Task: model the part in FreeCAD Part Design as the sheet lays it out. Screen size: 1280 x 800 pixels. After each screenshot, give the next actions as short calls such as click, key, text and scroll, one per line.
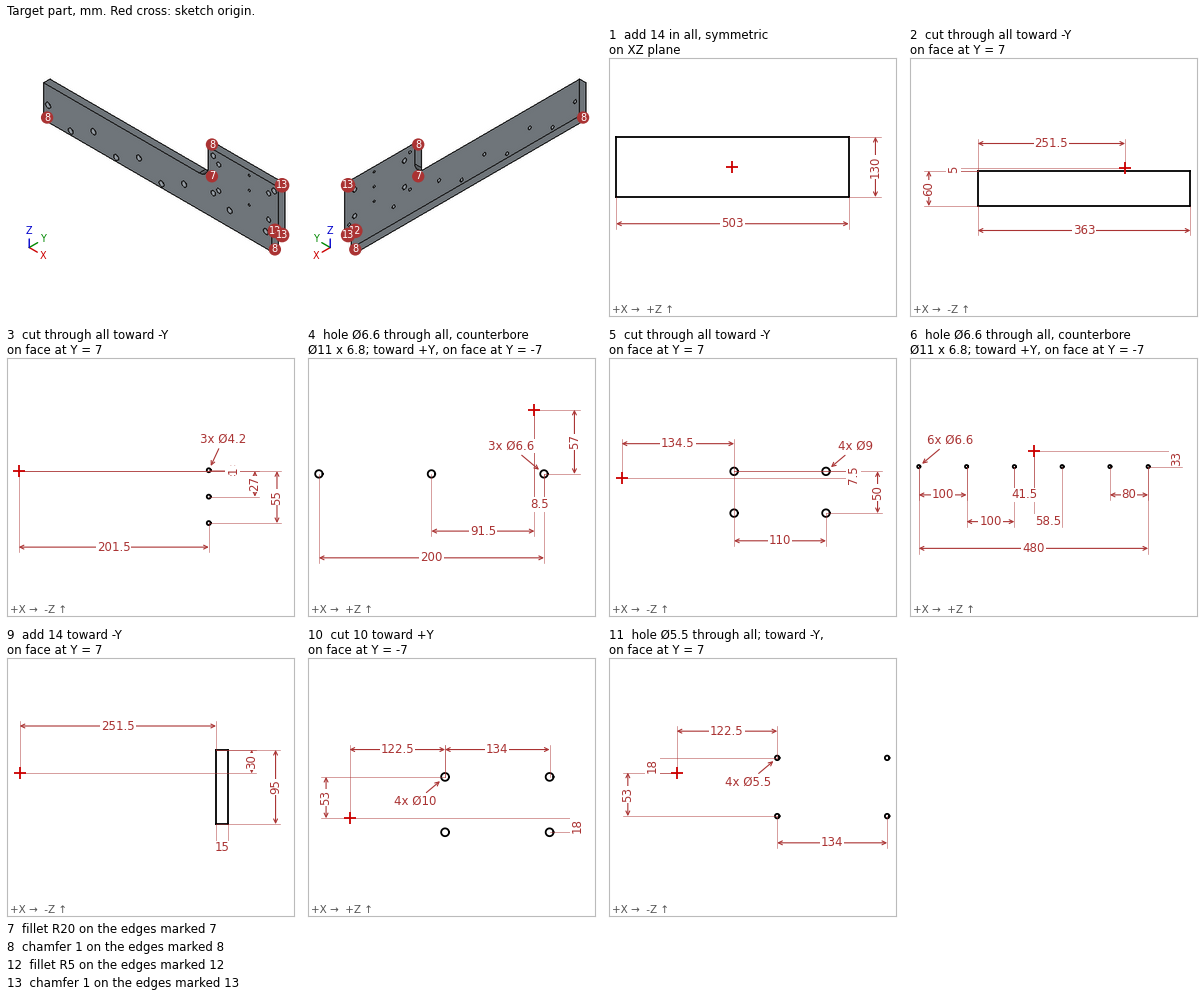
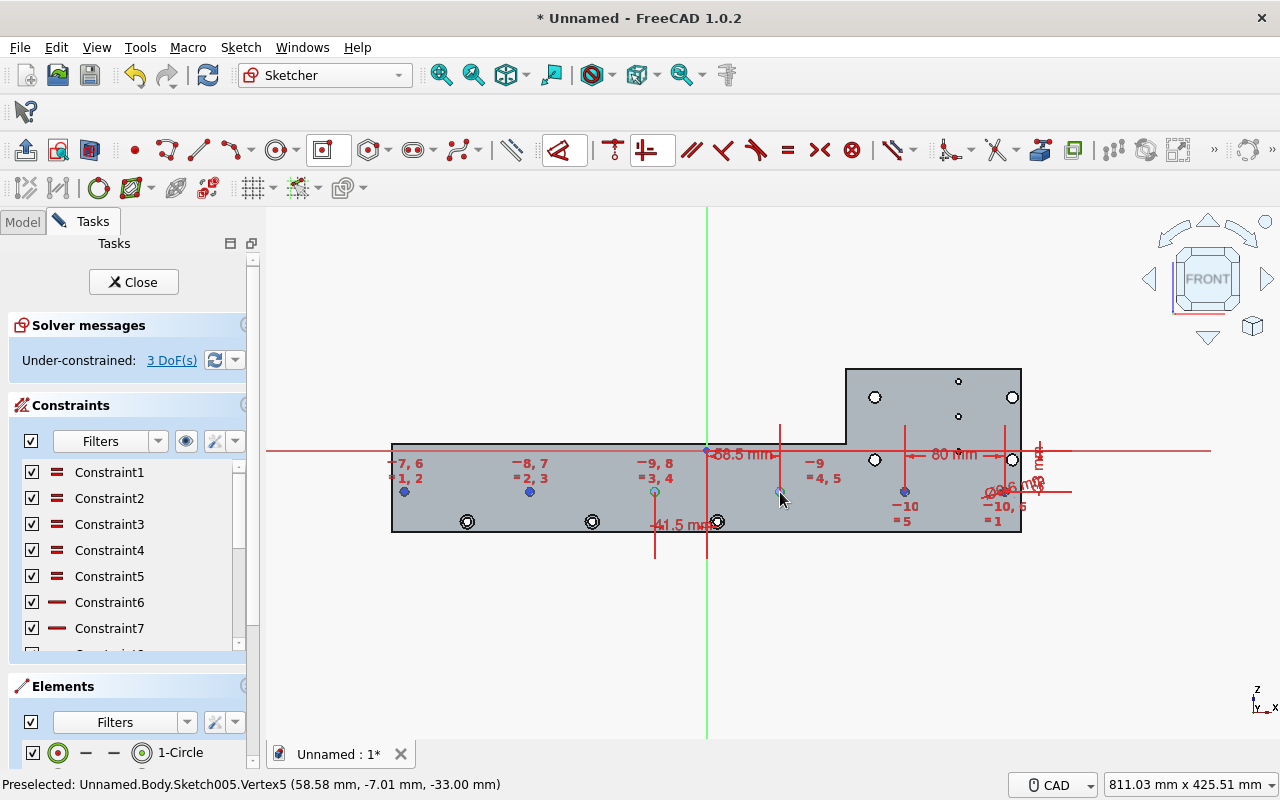
click(1005, 492)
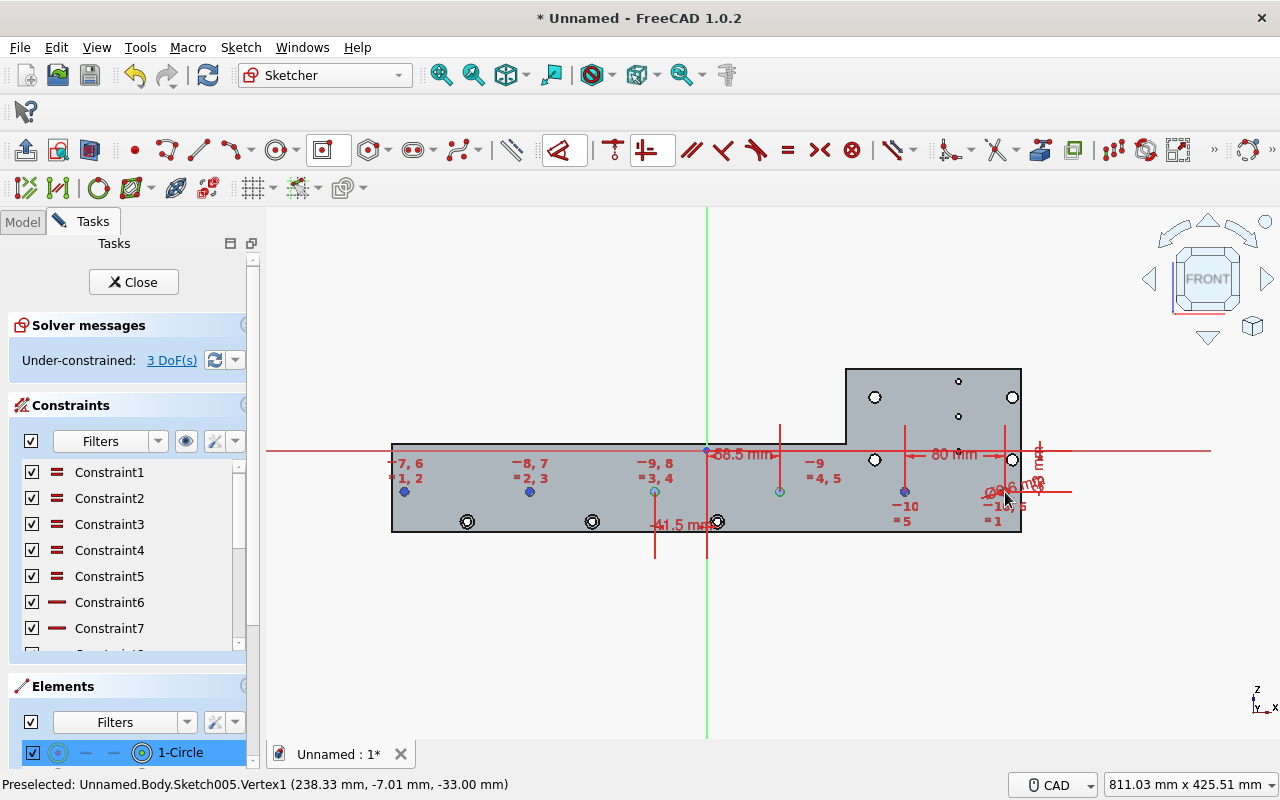
click(404, 492)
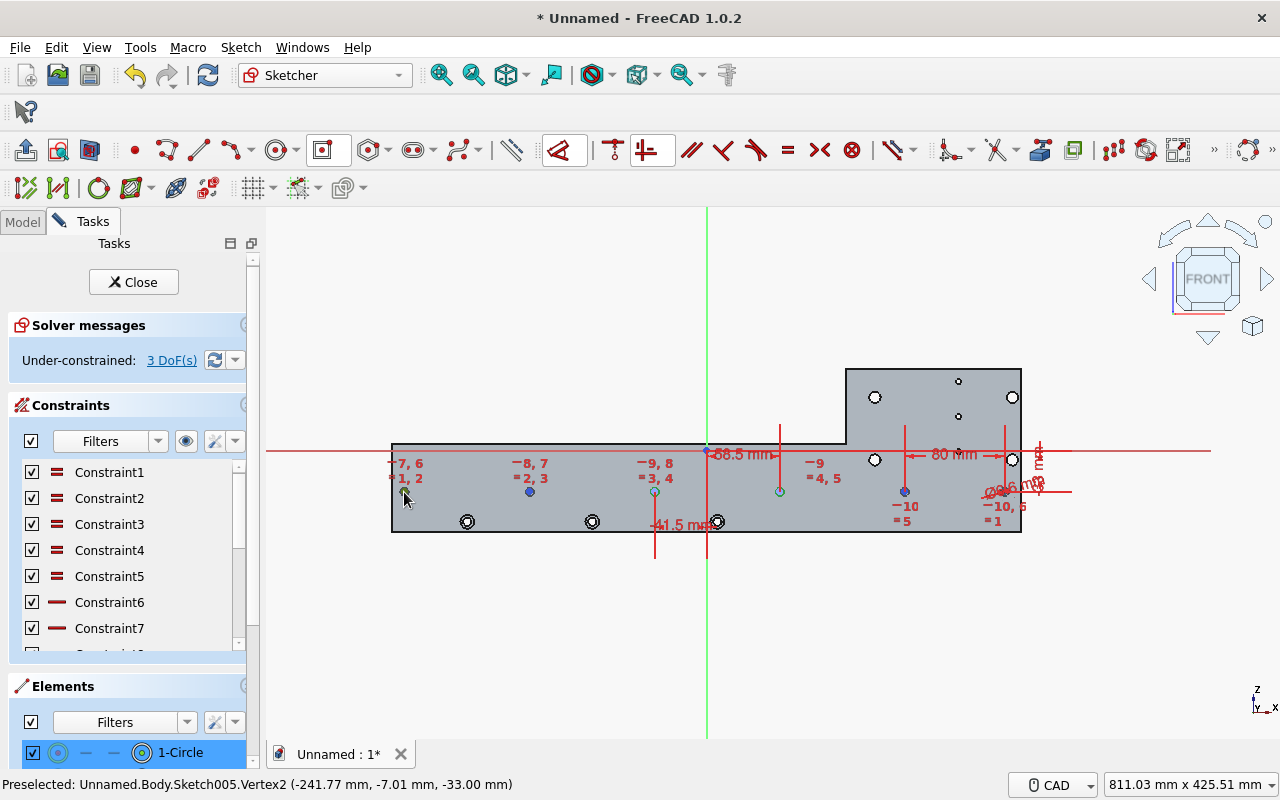
key(l)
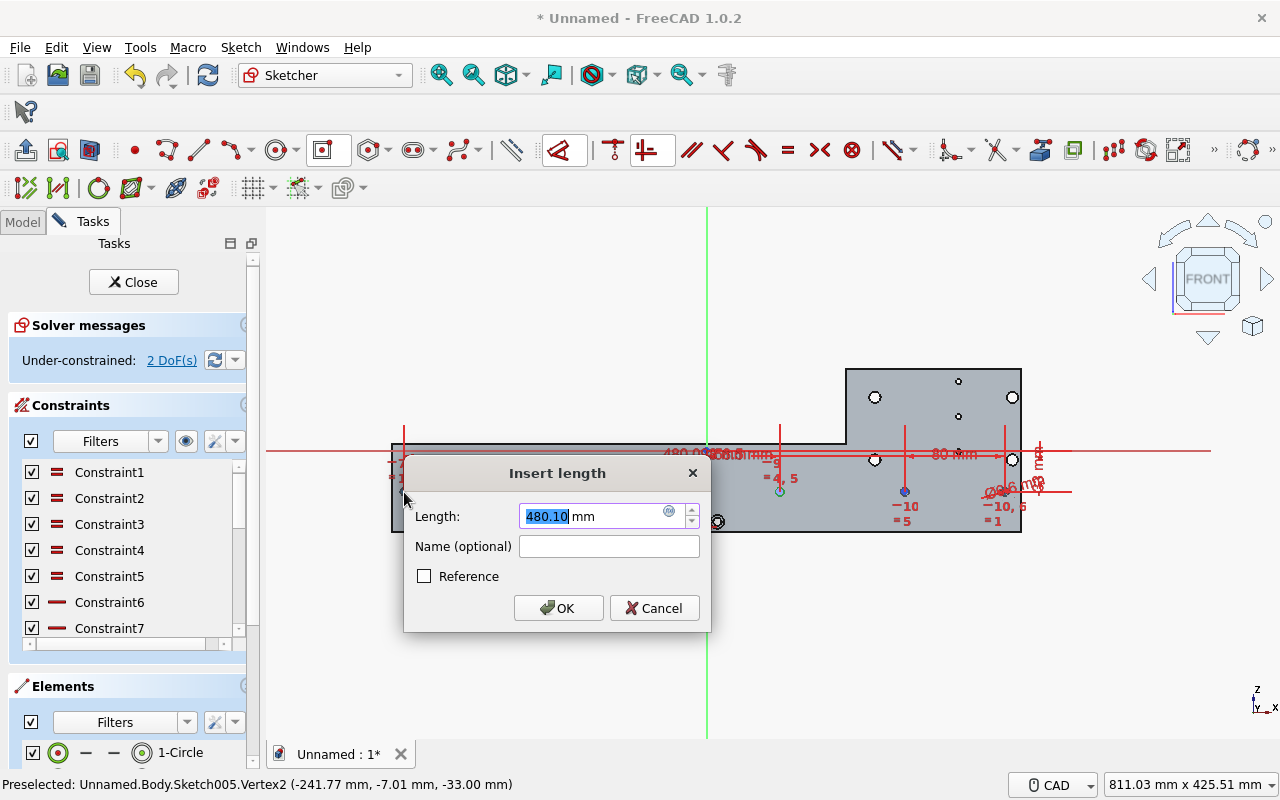
text(480)
key(Return)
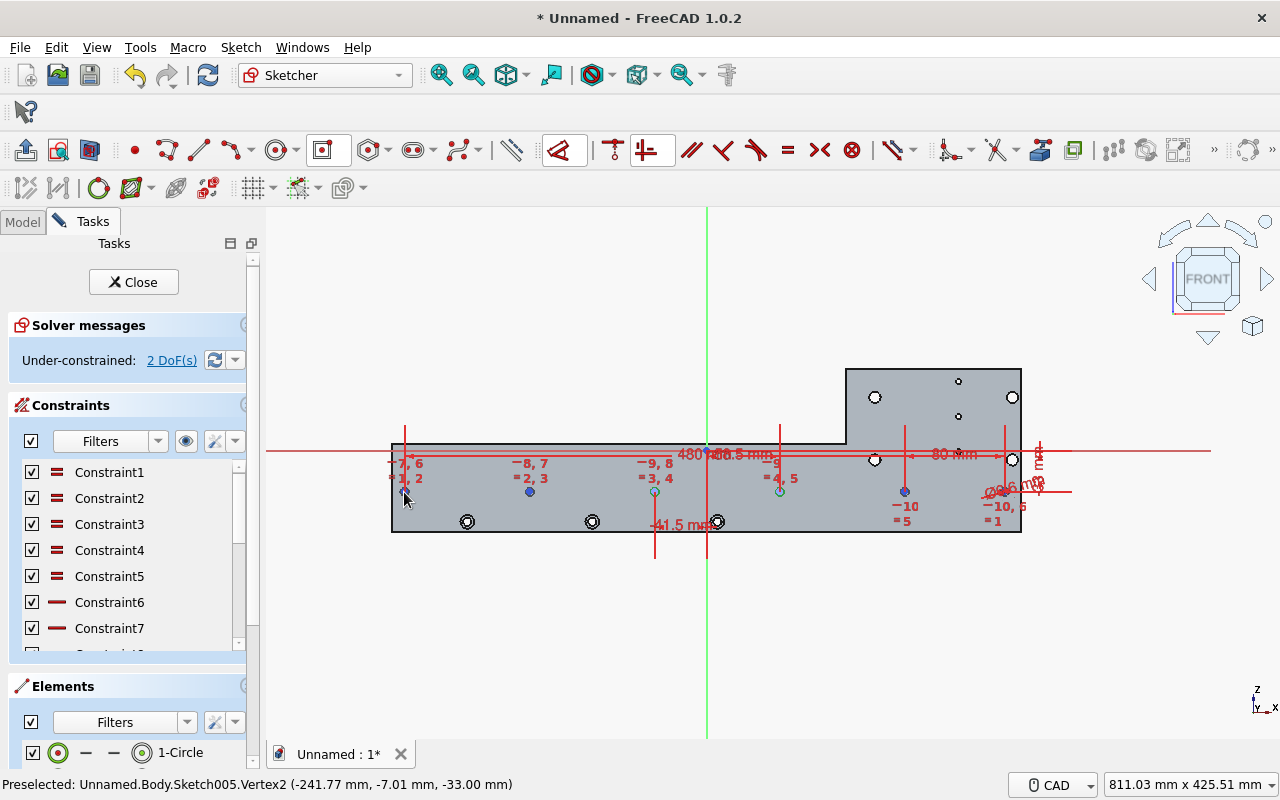
click(405, 492)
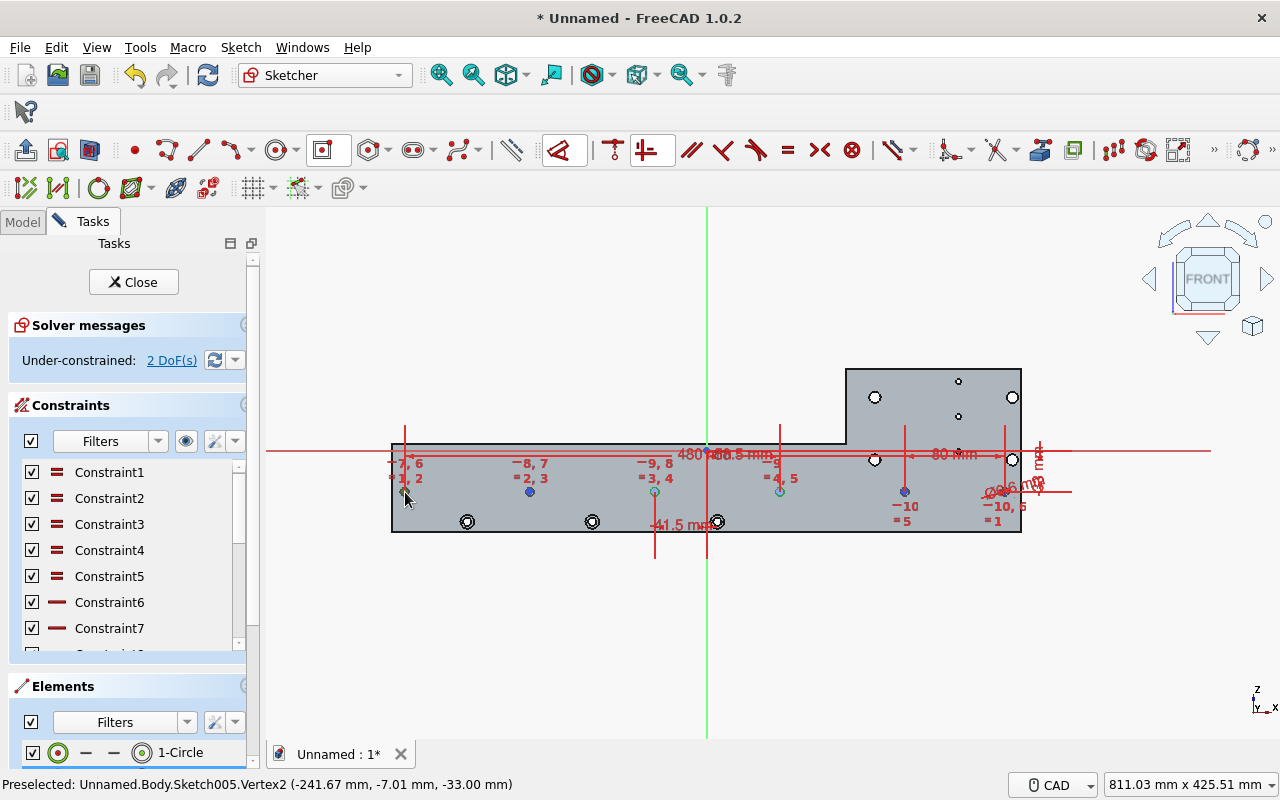
click(530, 492)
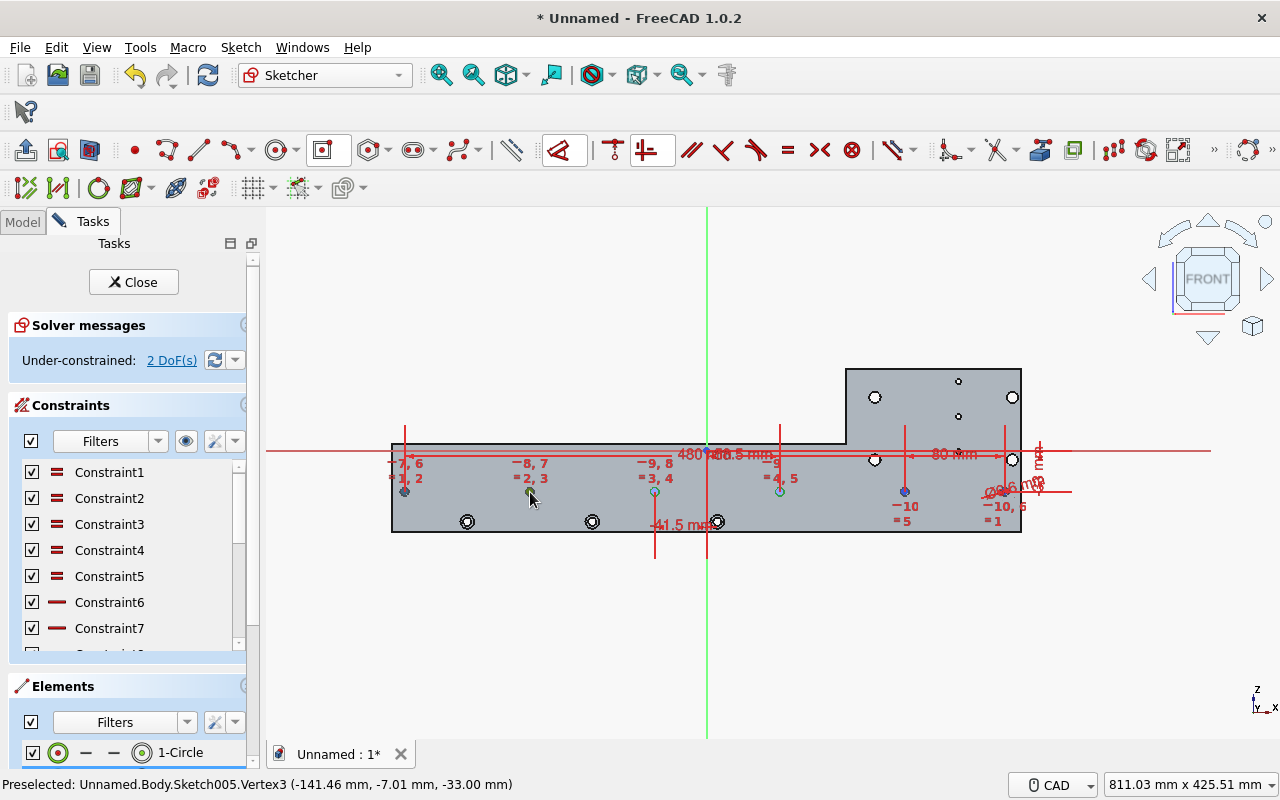
key(l)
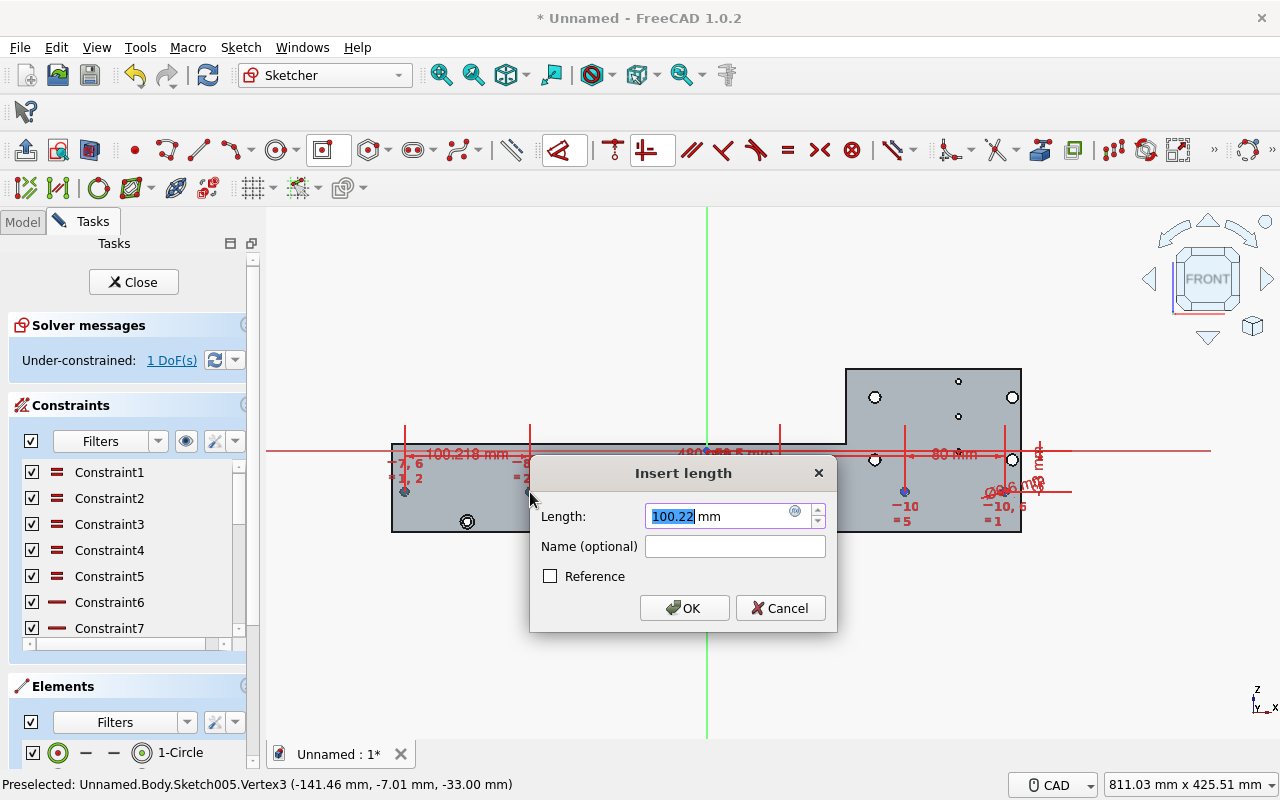
text(100)
key(Return)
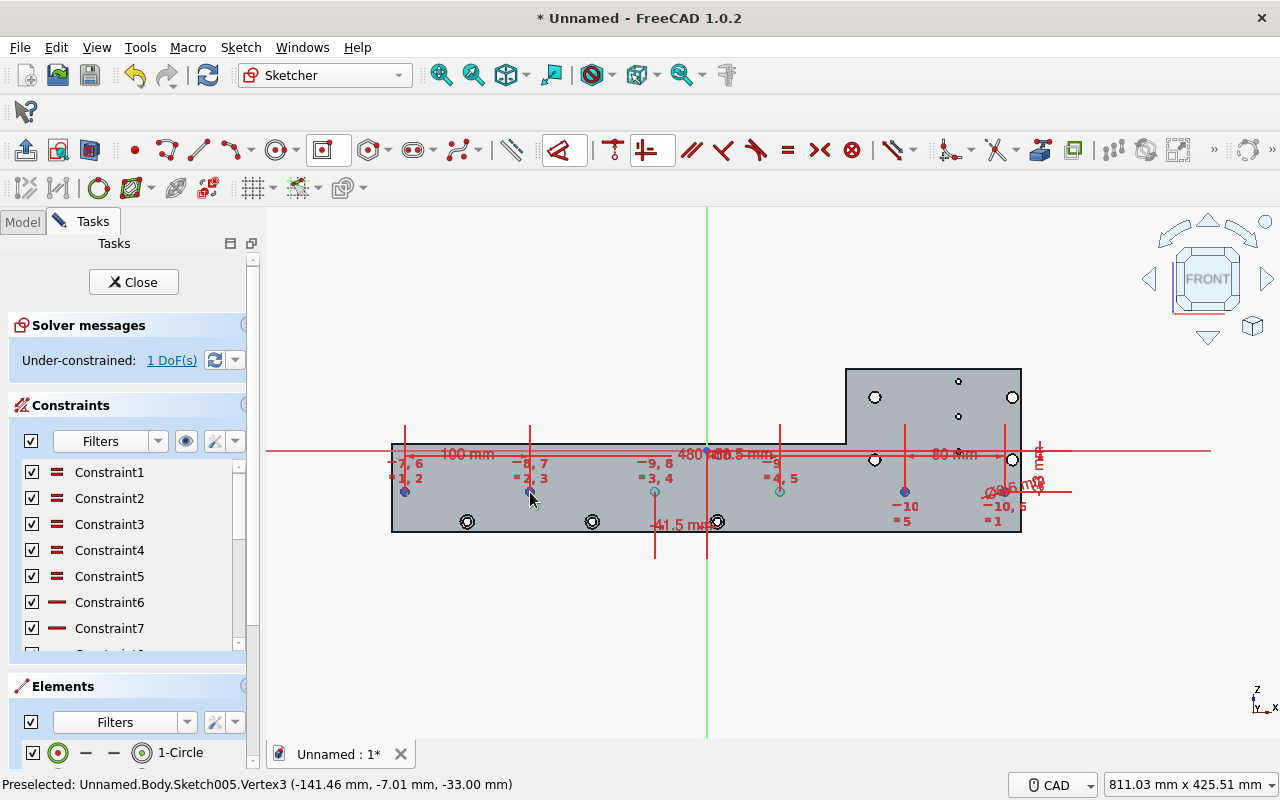
click(530, 492)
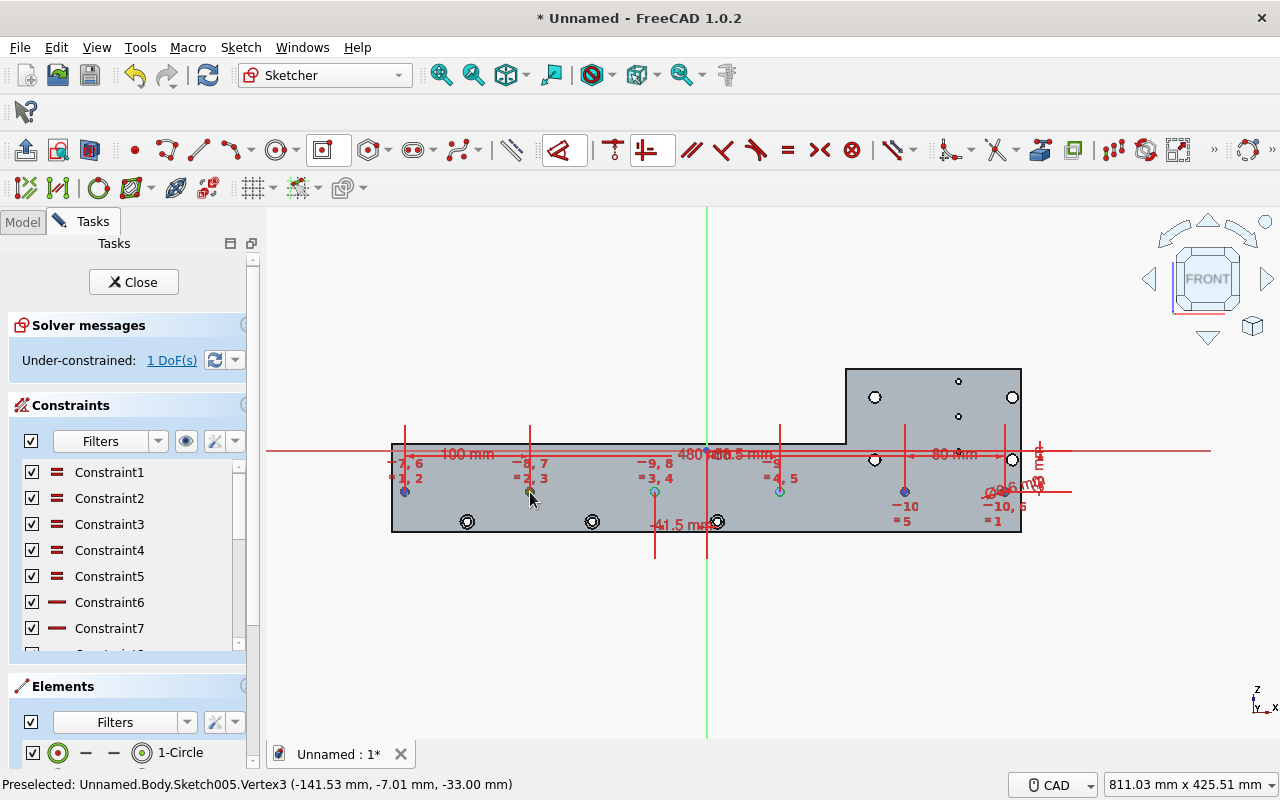
click(655, 492)